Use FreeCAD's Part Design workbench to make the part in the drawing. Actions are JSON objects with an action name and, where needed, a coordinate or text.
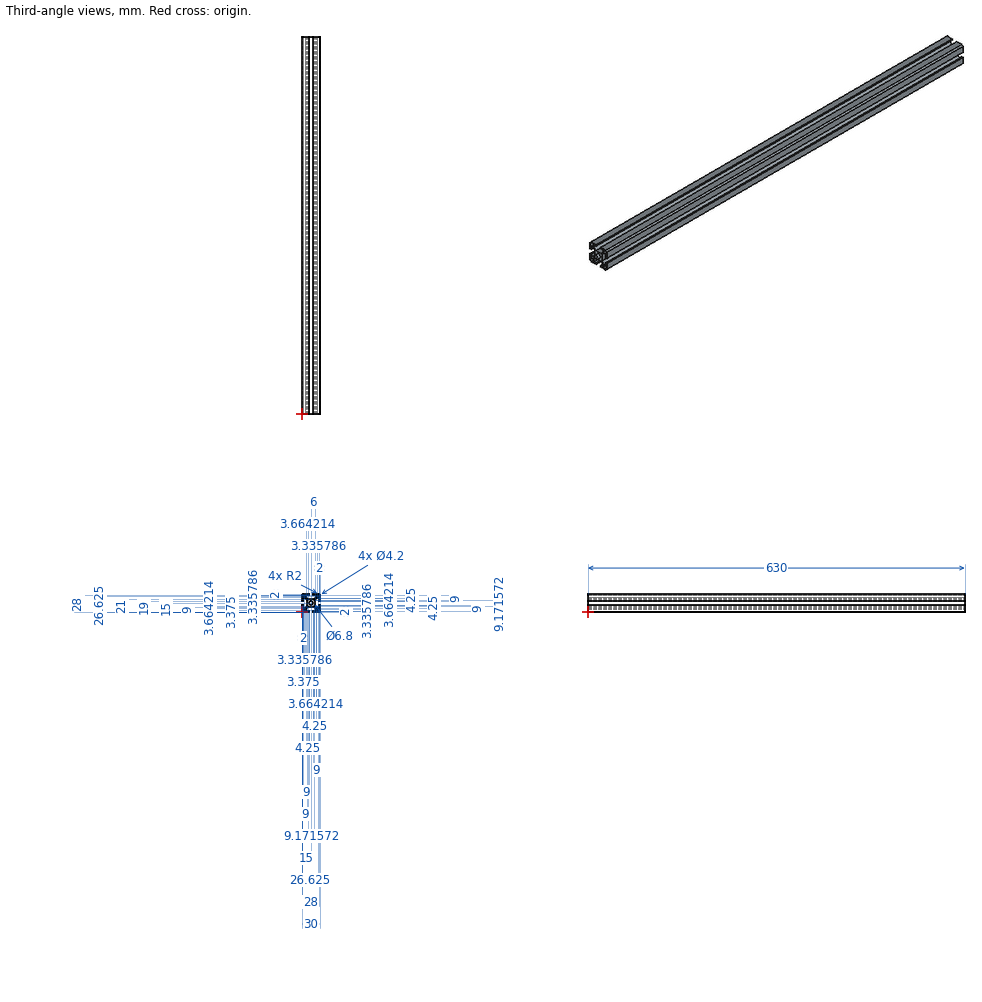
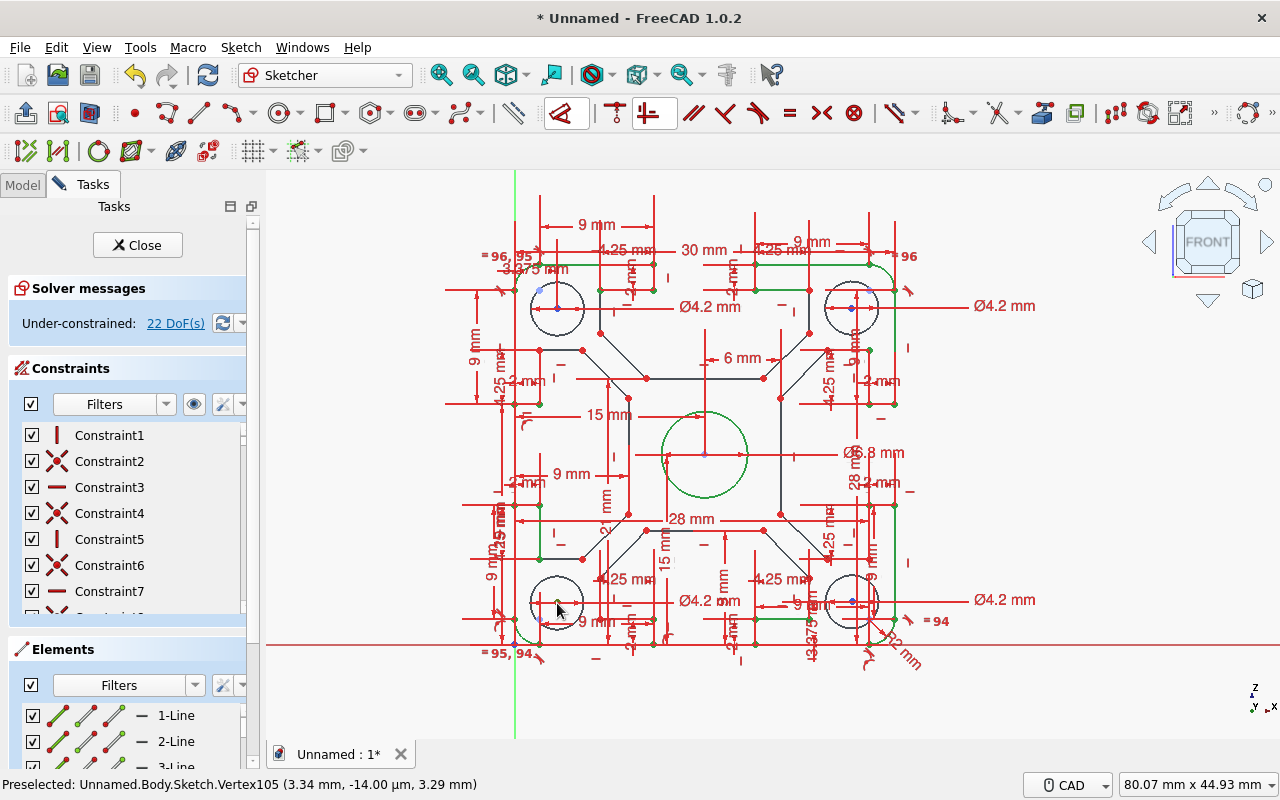
{"action": "left_click", "coordinate": [584, 114]}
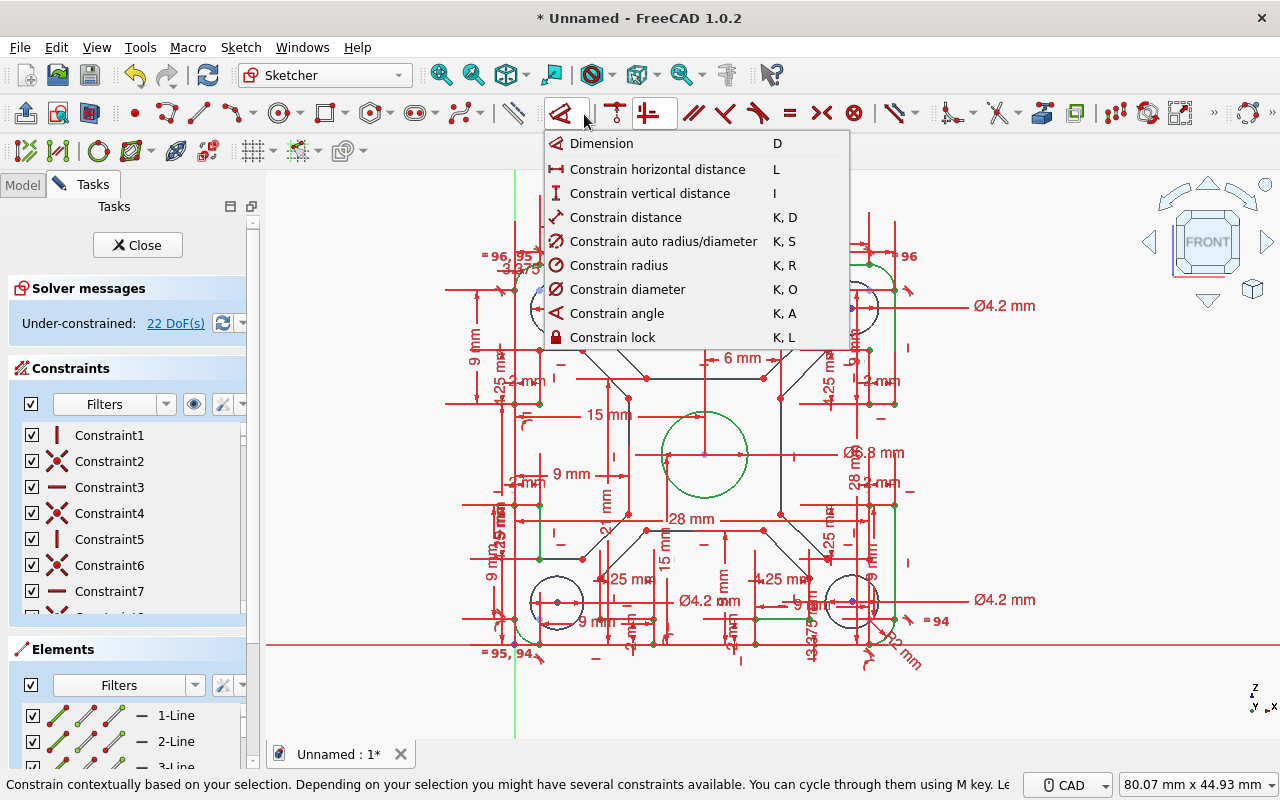
{"action": "left_click", "coordinate": [697, 169]}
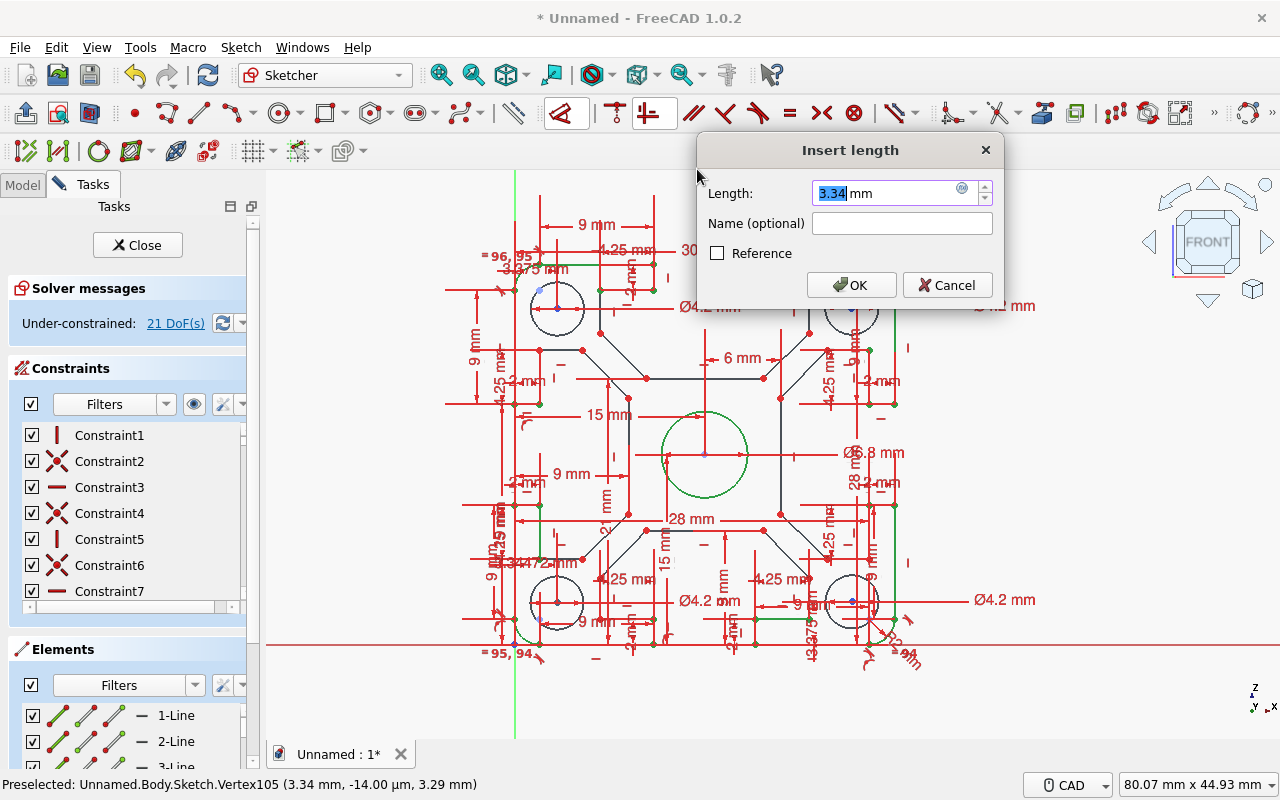
{"action": "type", "text": "3.375"}
{"action": "key", "text": "Return"}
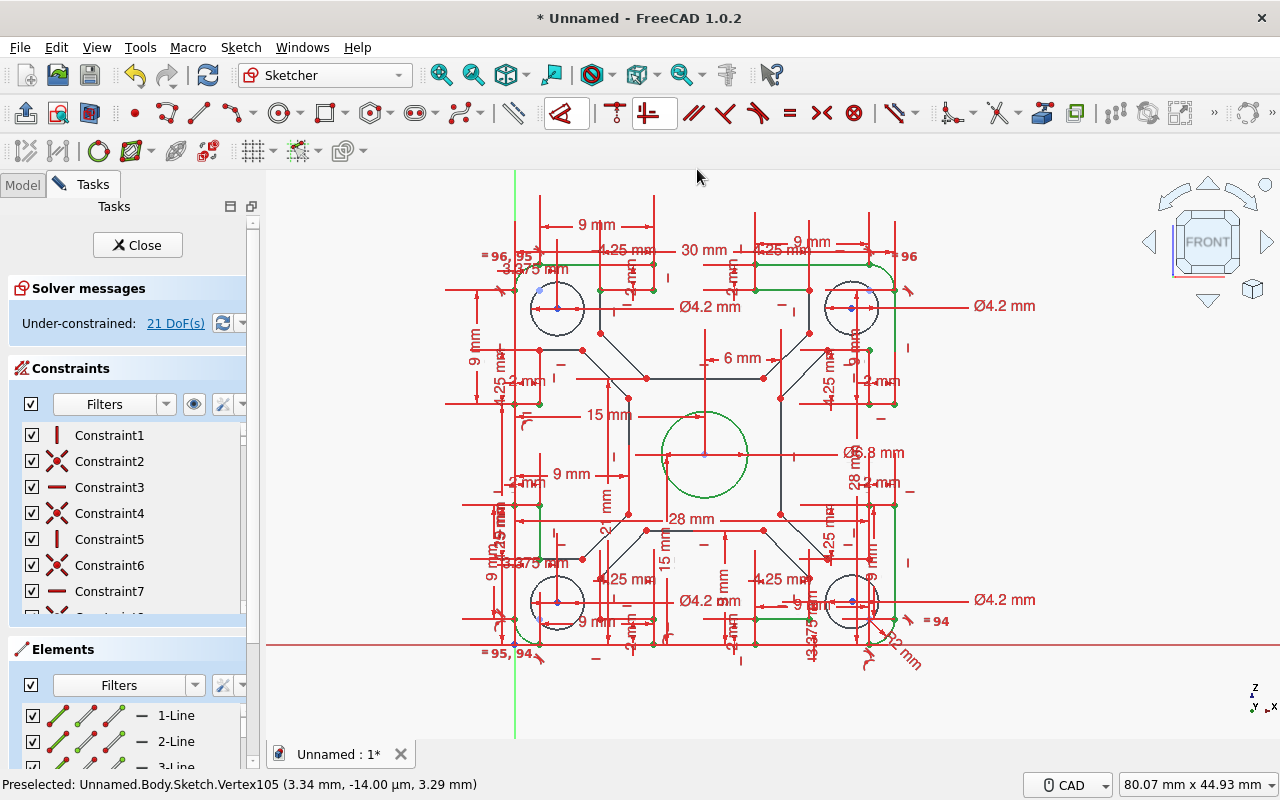
{"action": "left_click", "coordinate": [557, 603]}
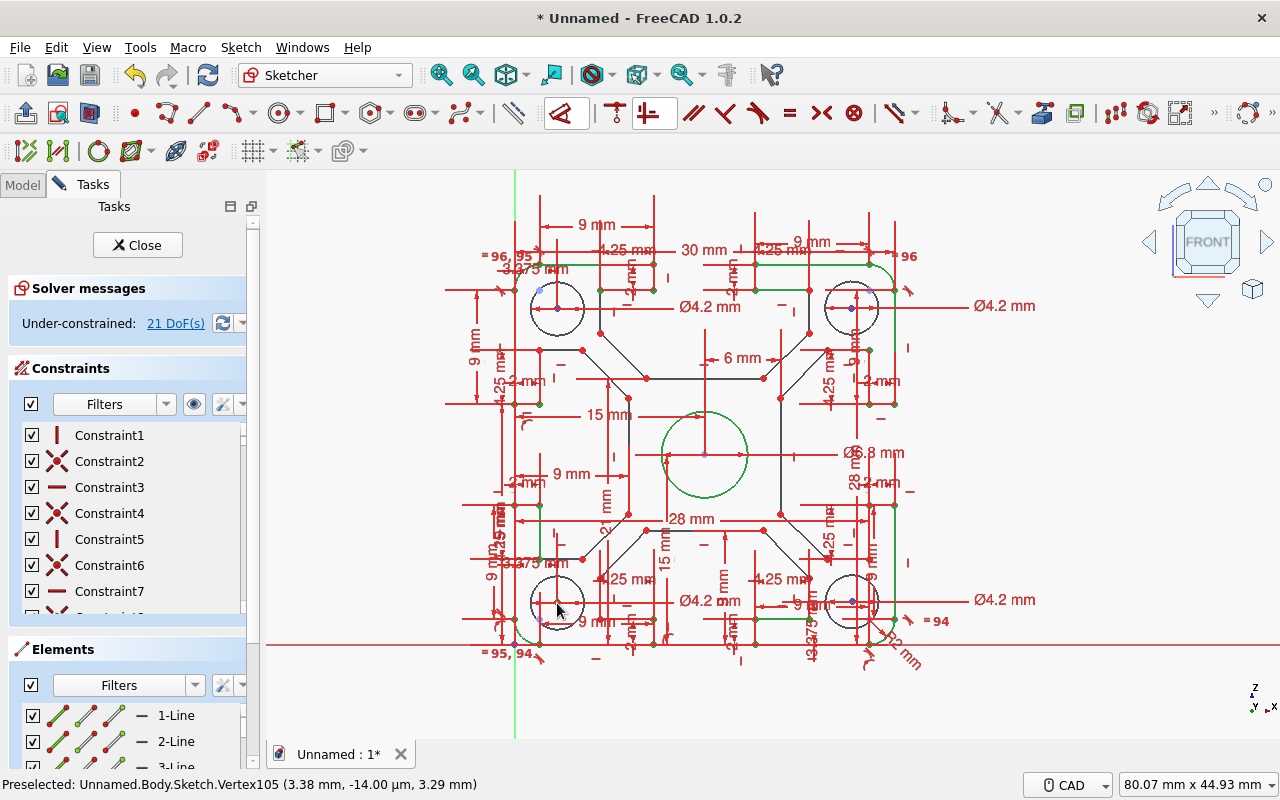
{"action": "left_click", "coordinate": [584, 114]}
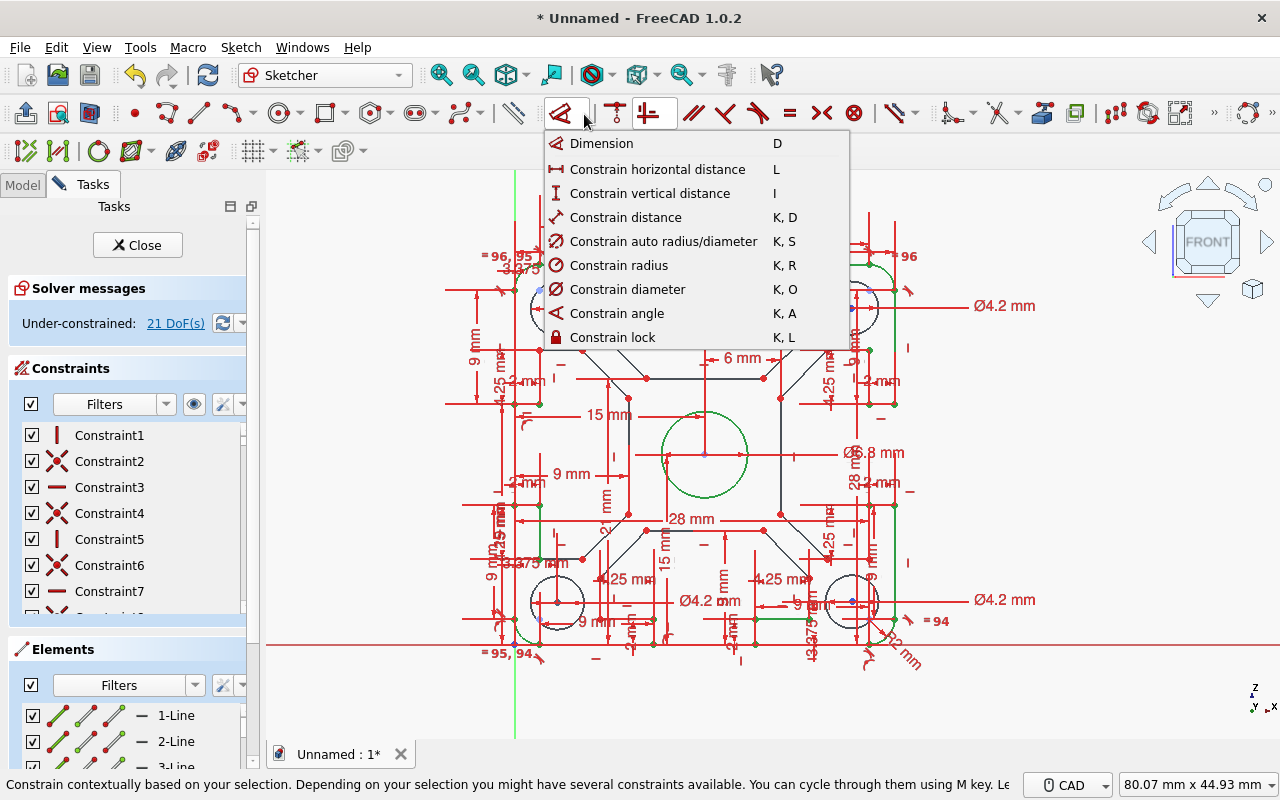
{"action": "left_click", "coordinate": [697, 193]}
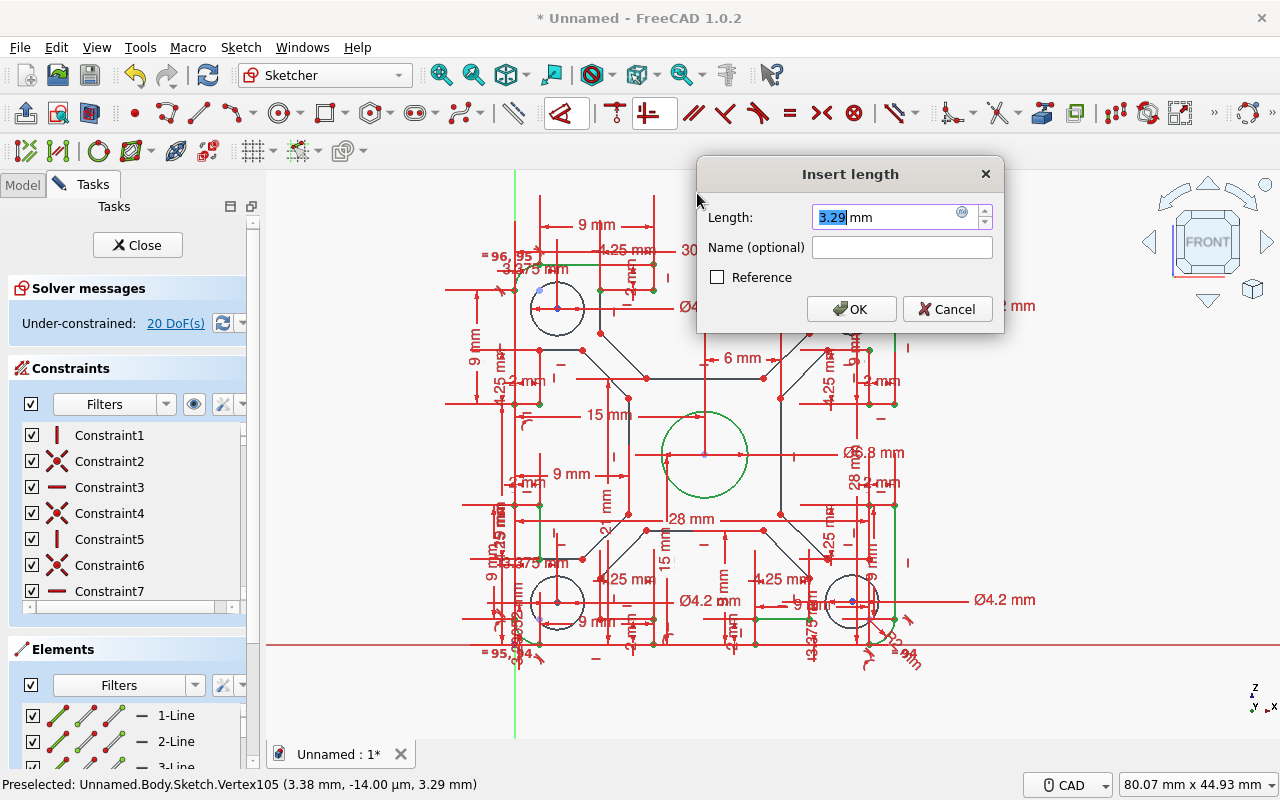
{"action": "type", "text": "3.375"}
{"action": "key", "text": "Return"}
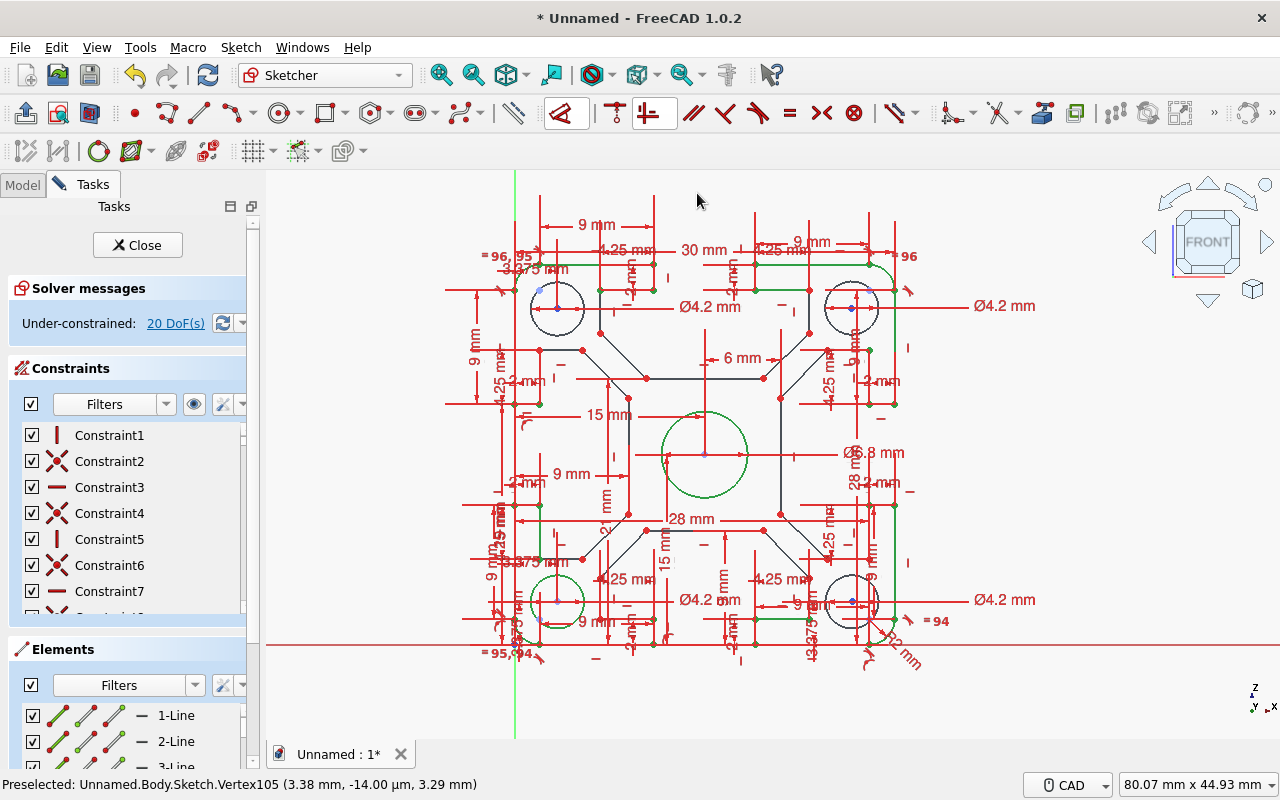
{"action": "left_click", "coordinate": [852, 308]}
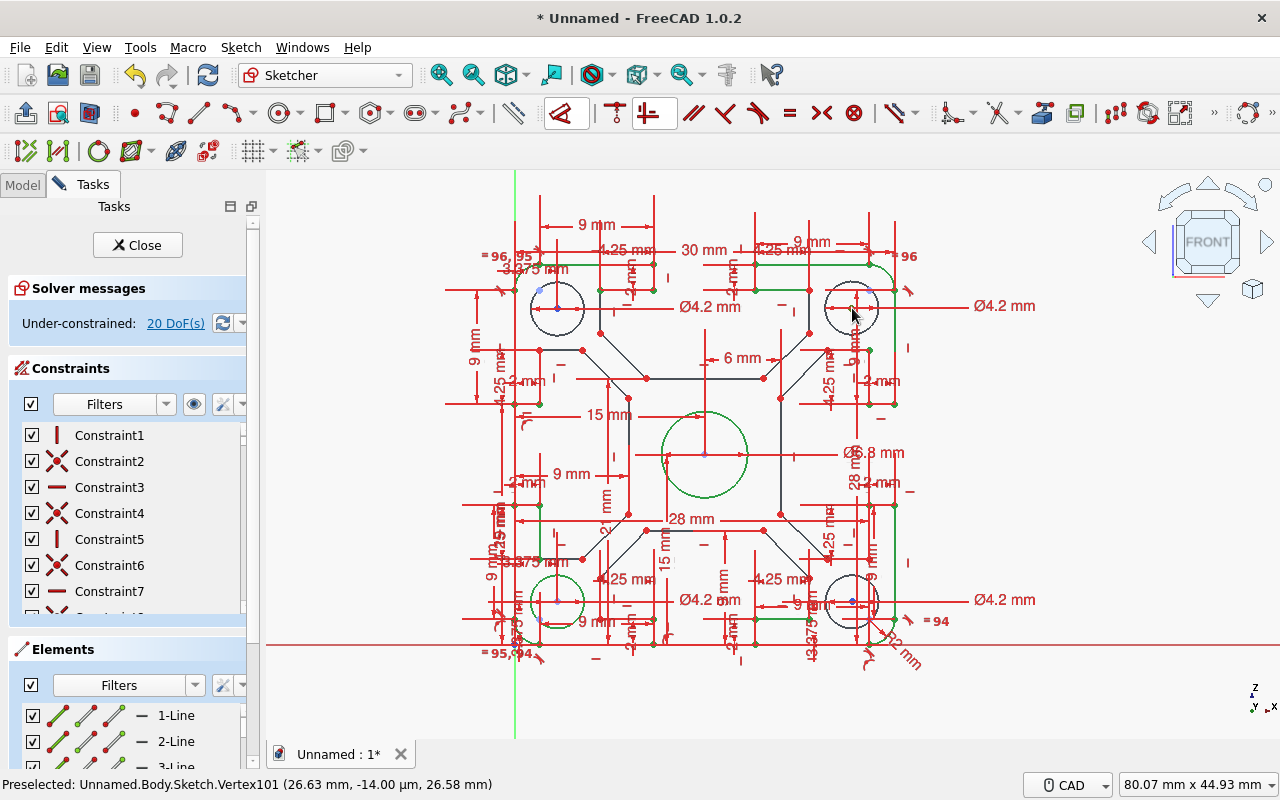
{"action": "key", "text": "l"}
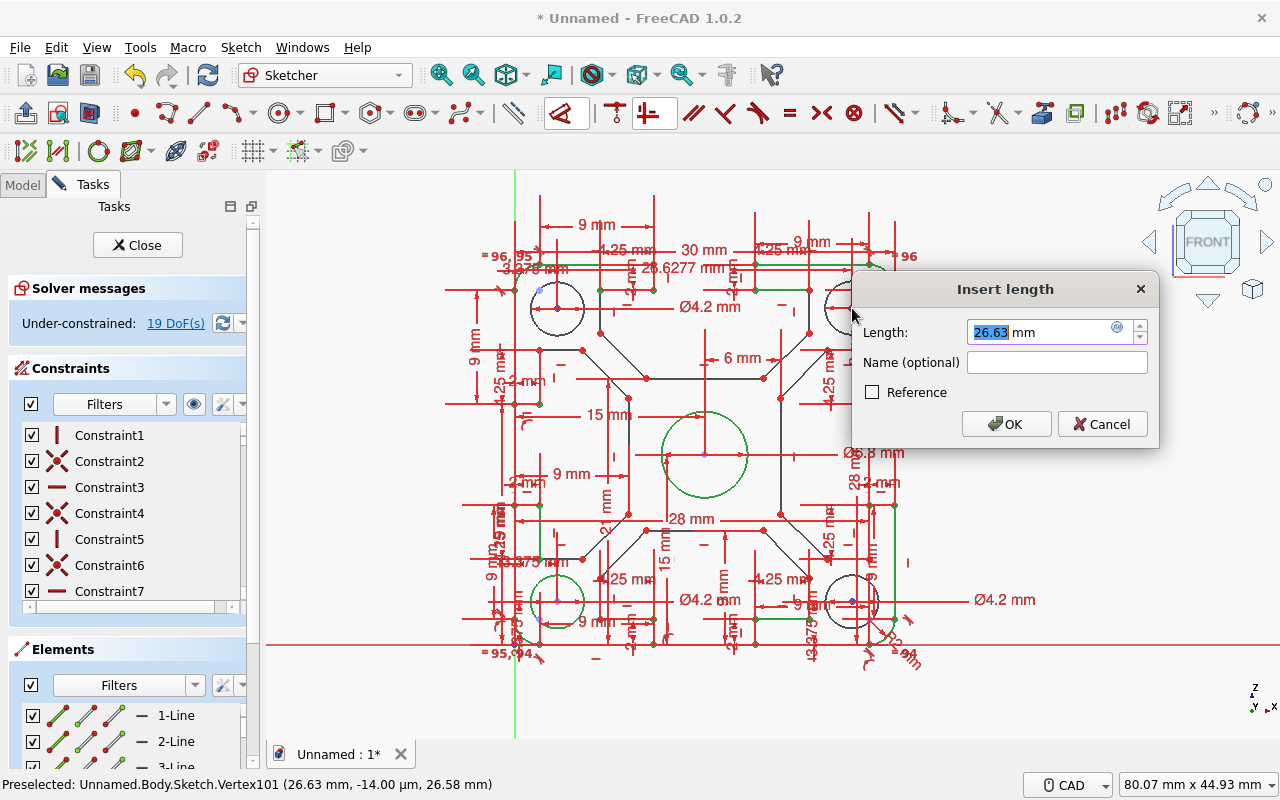
{"action": "type", "text": "26.625"}
{"action": "key", "text": "Return"}